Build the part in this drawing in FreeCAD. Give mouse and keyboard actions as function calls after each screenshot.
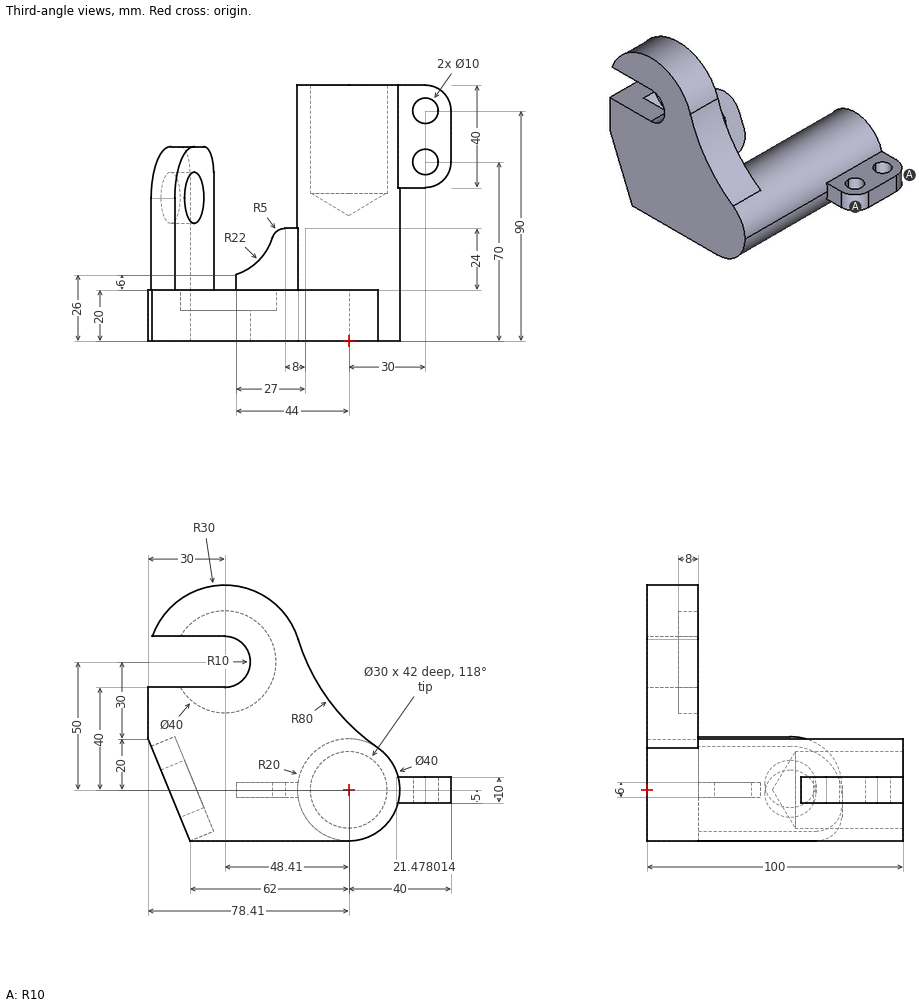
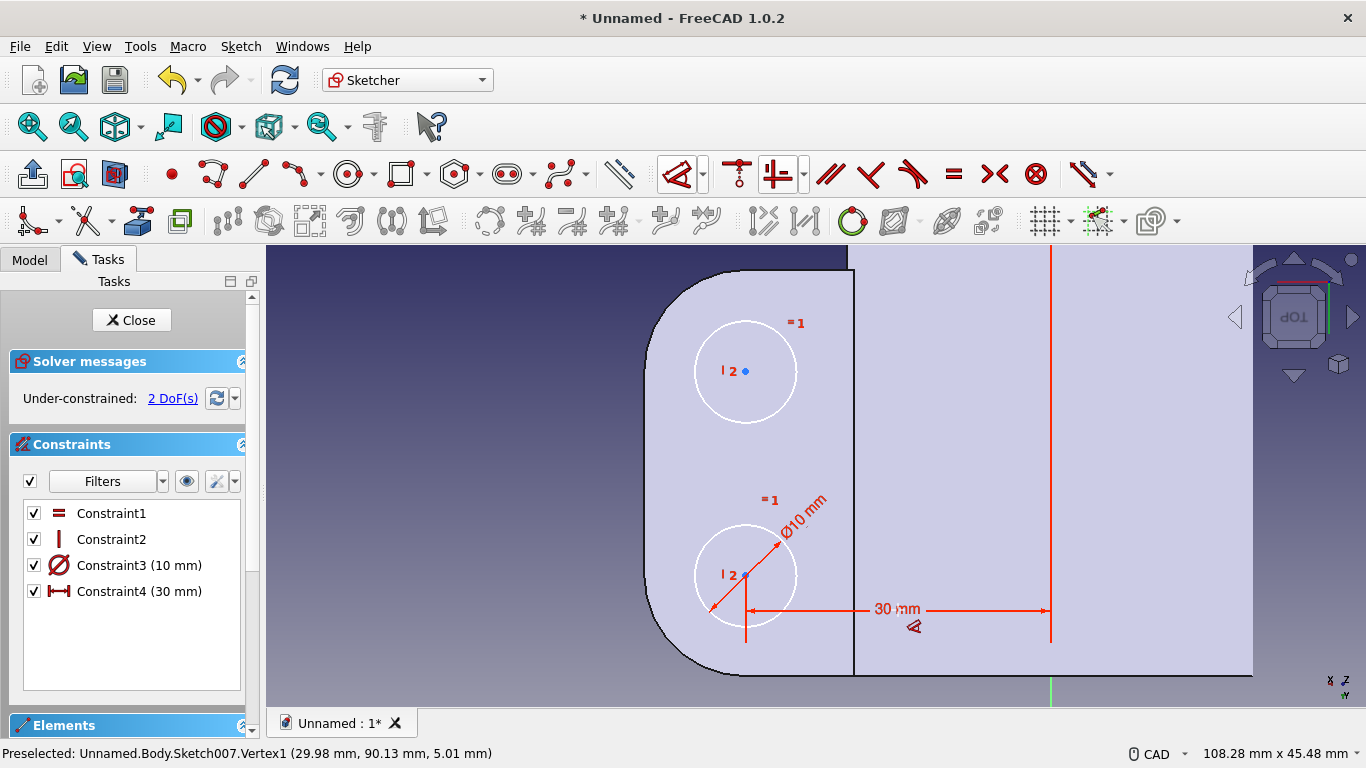
click(746, 576)
click(1085, 424)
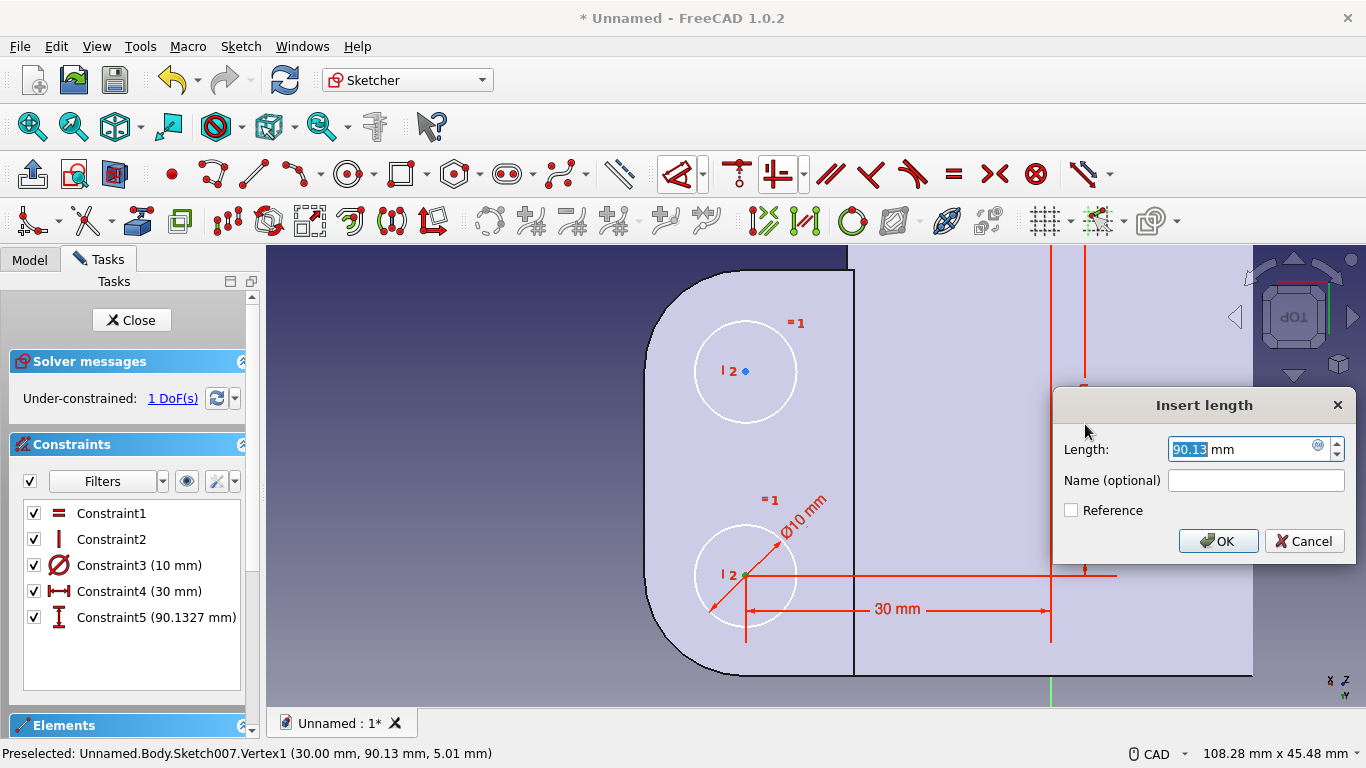
text(90)
key(Return)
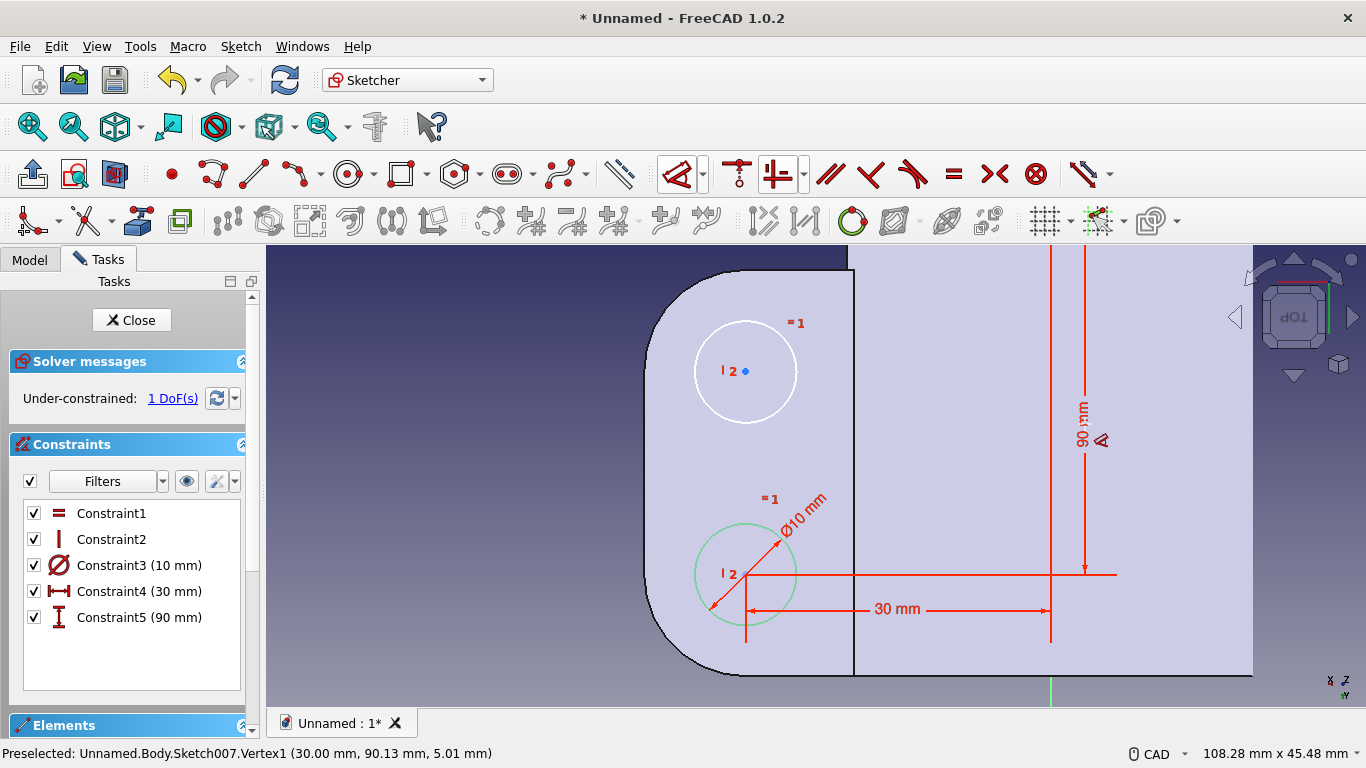
click(746, 372)
click(1085, 322)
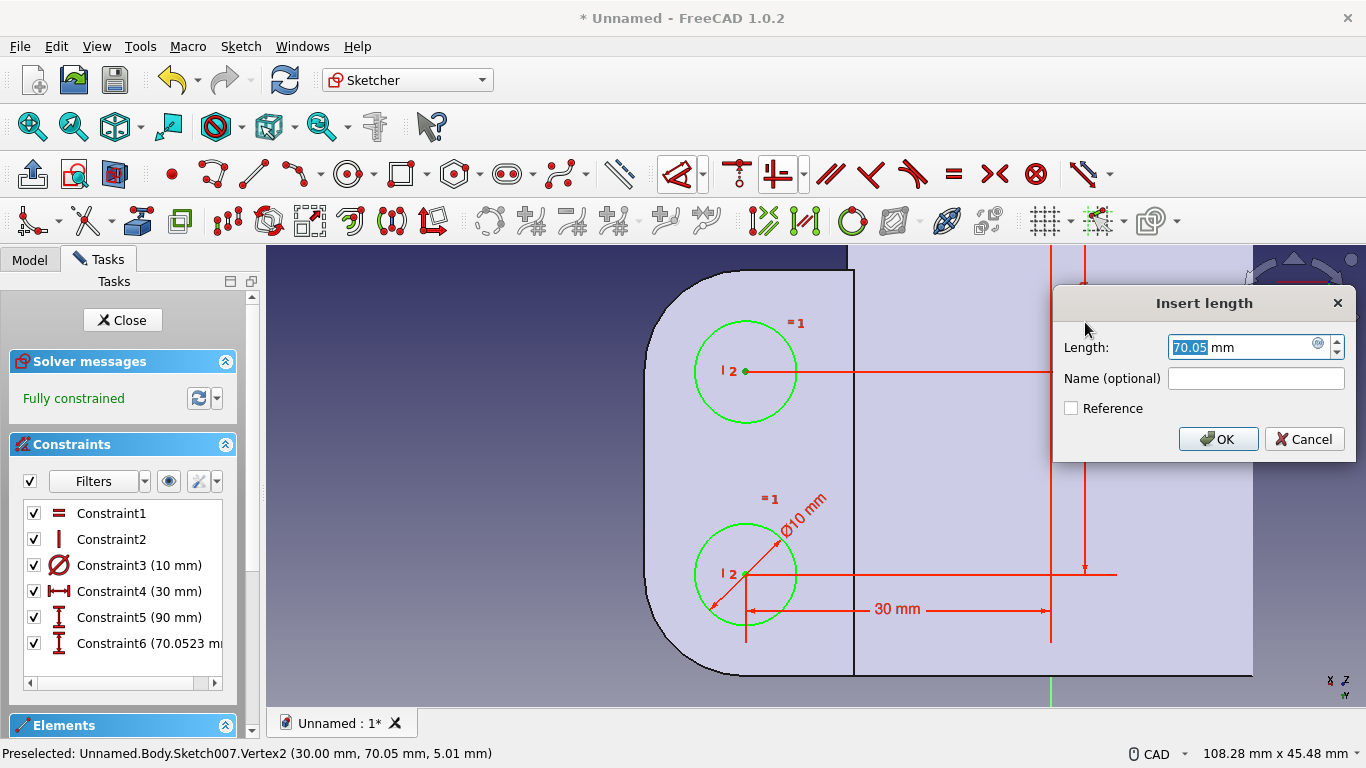
text(70)
key(Return)
key(Escape)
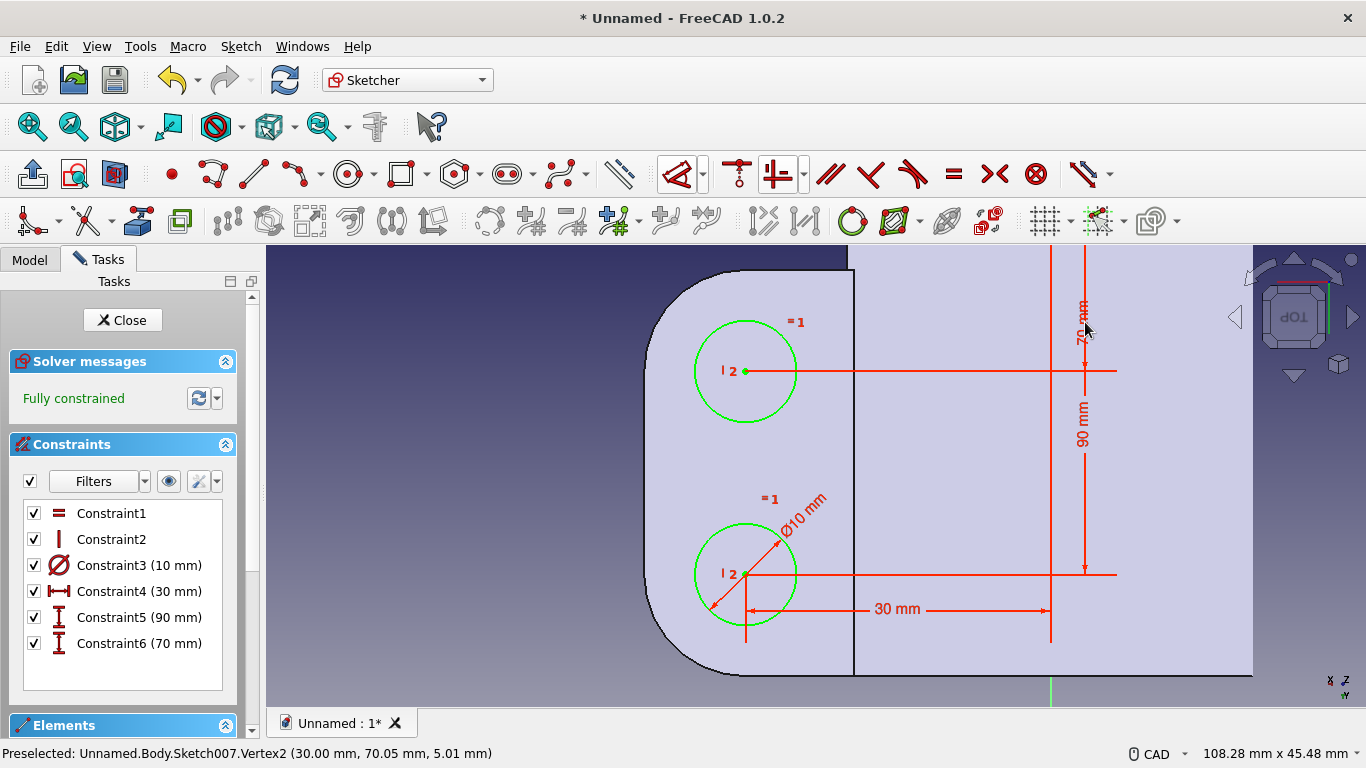
click(123, 320)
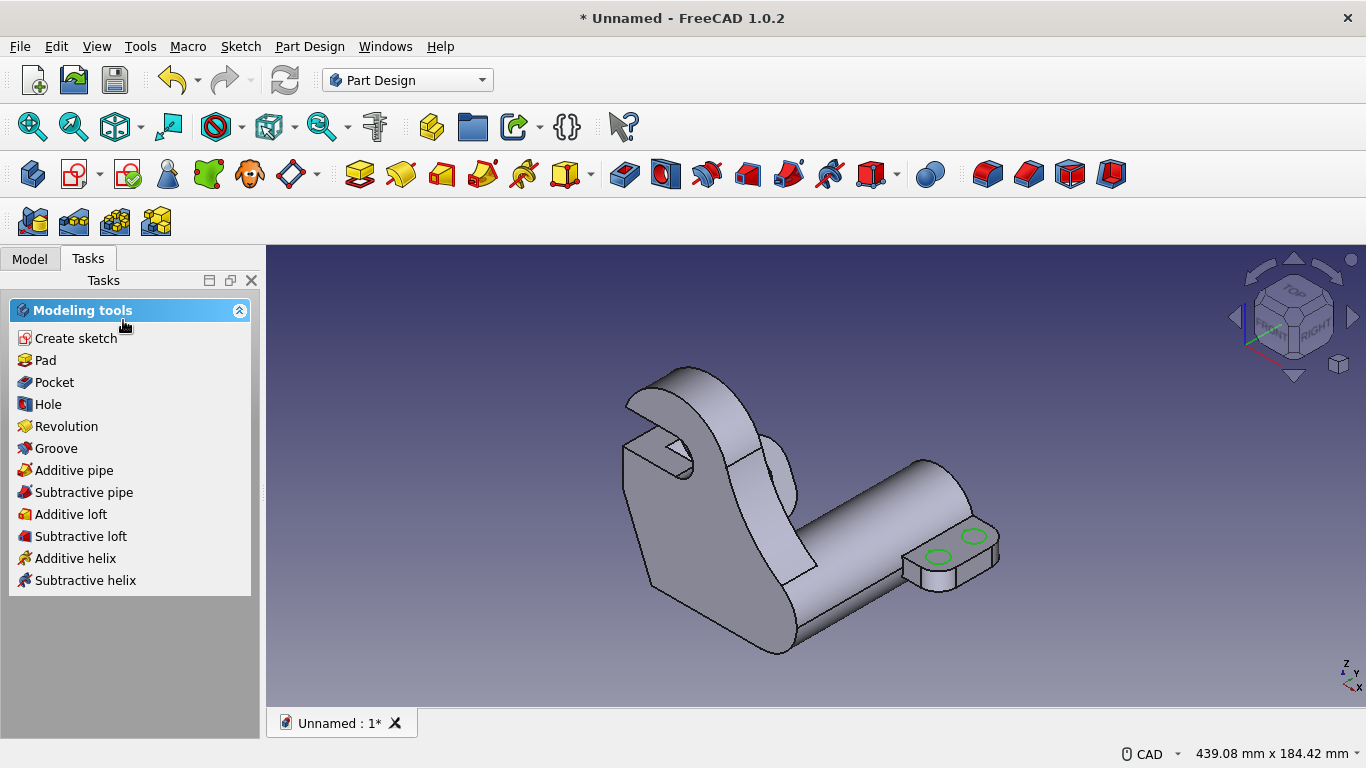
click(625, 174)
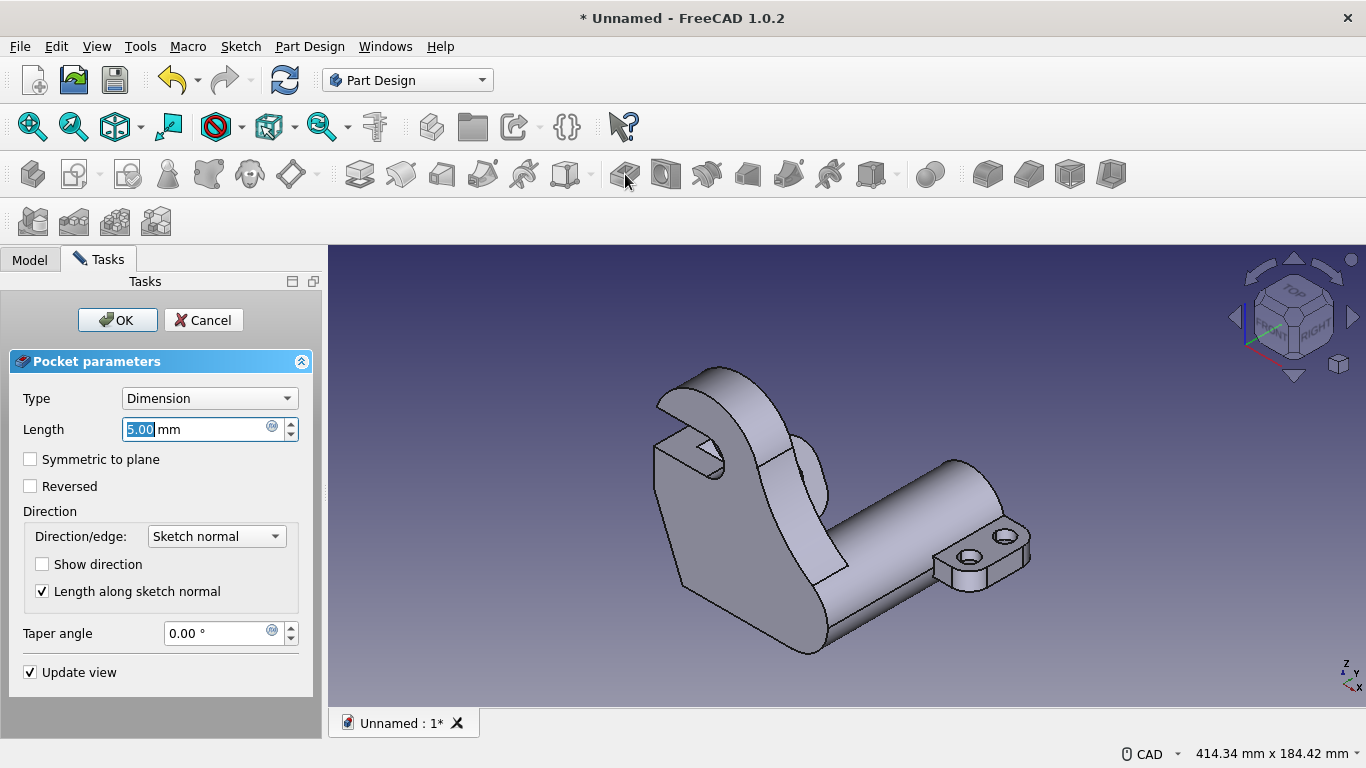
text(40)
key(Tab)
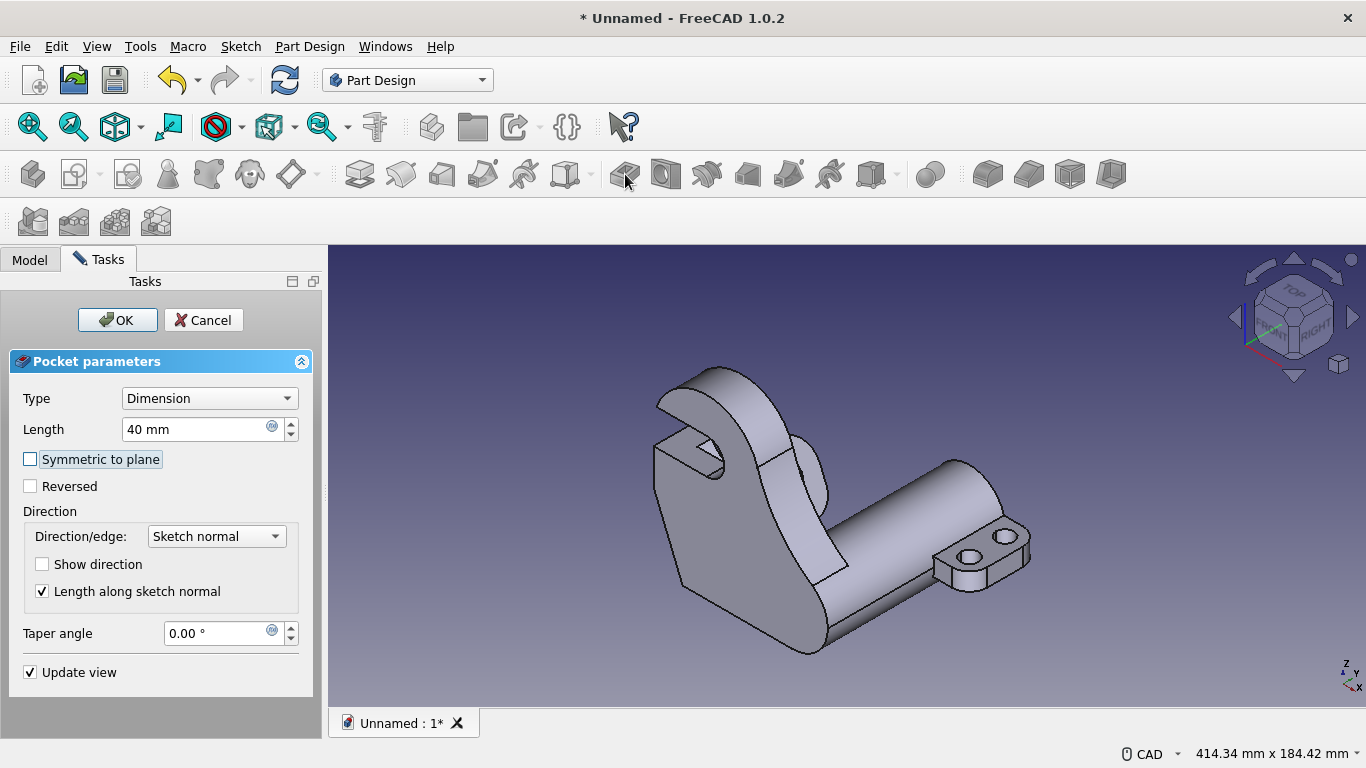
click(118, 320)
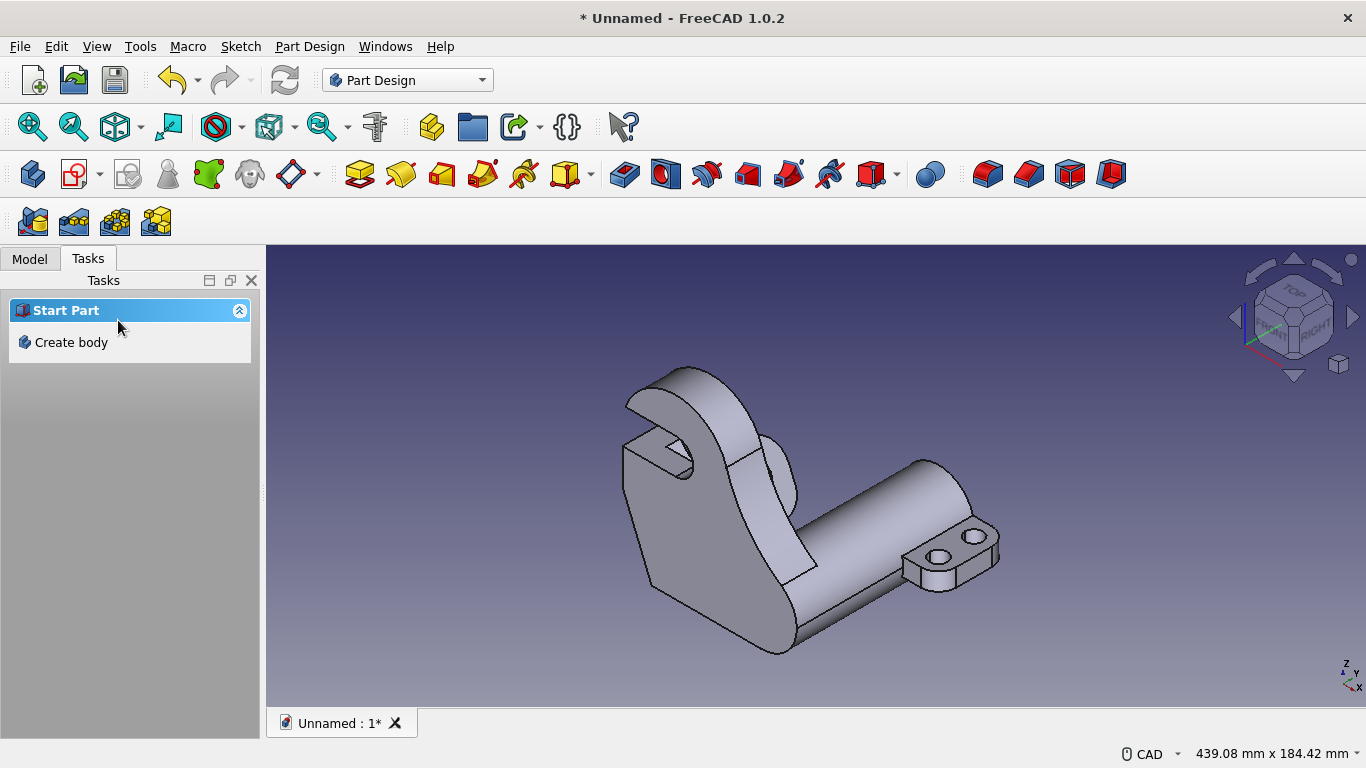
click(74, 174)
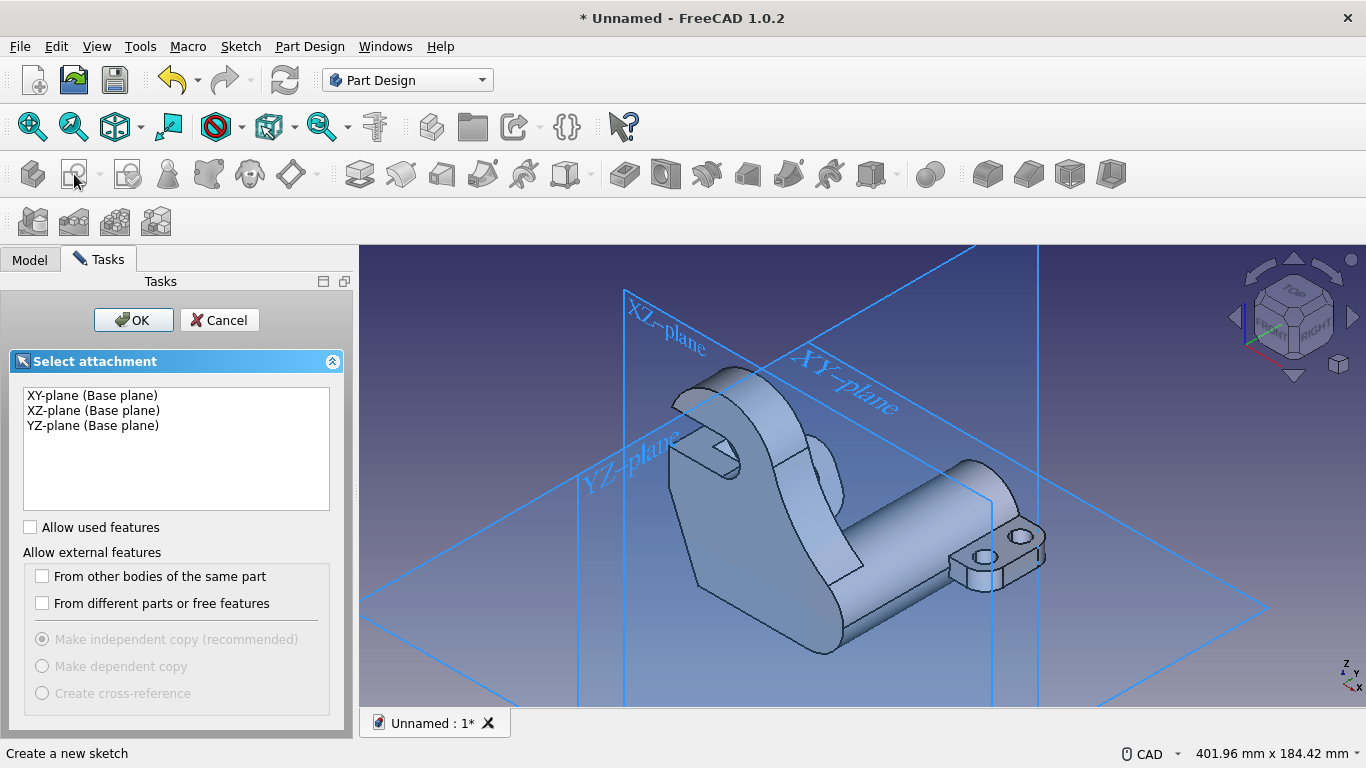
click(84, 396)